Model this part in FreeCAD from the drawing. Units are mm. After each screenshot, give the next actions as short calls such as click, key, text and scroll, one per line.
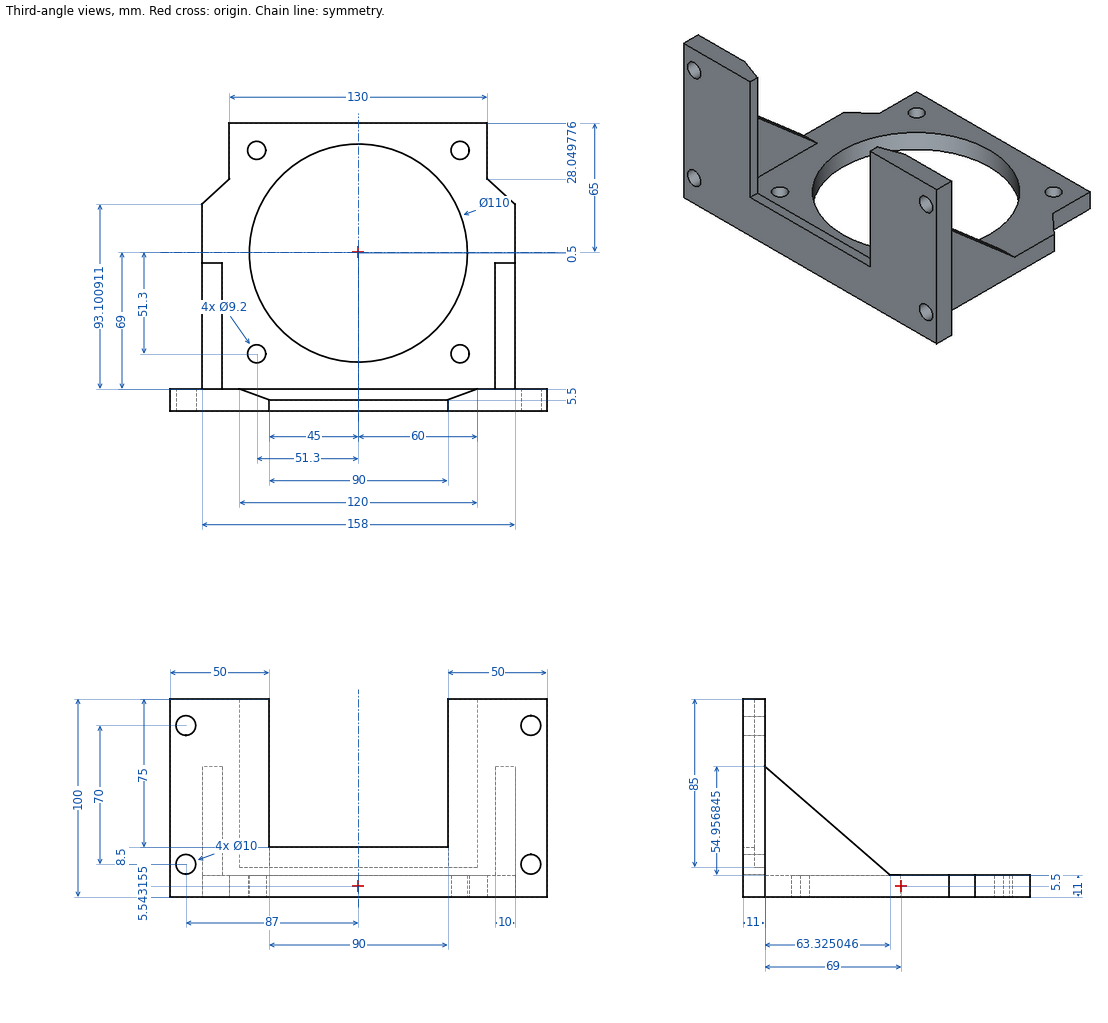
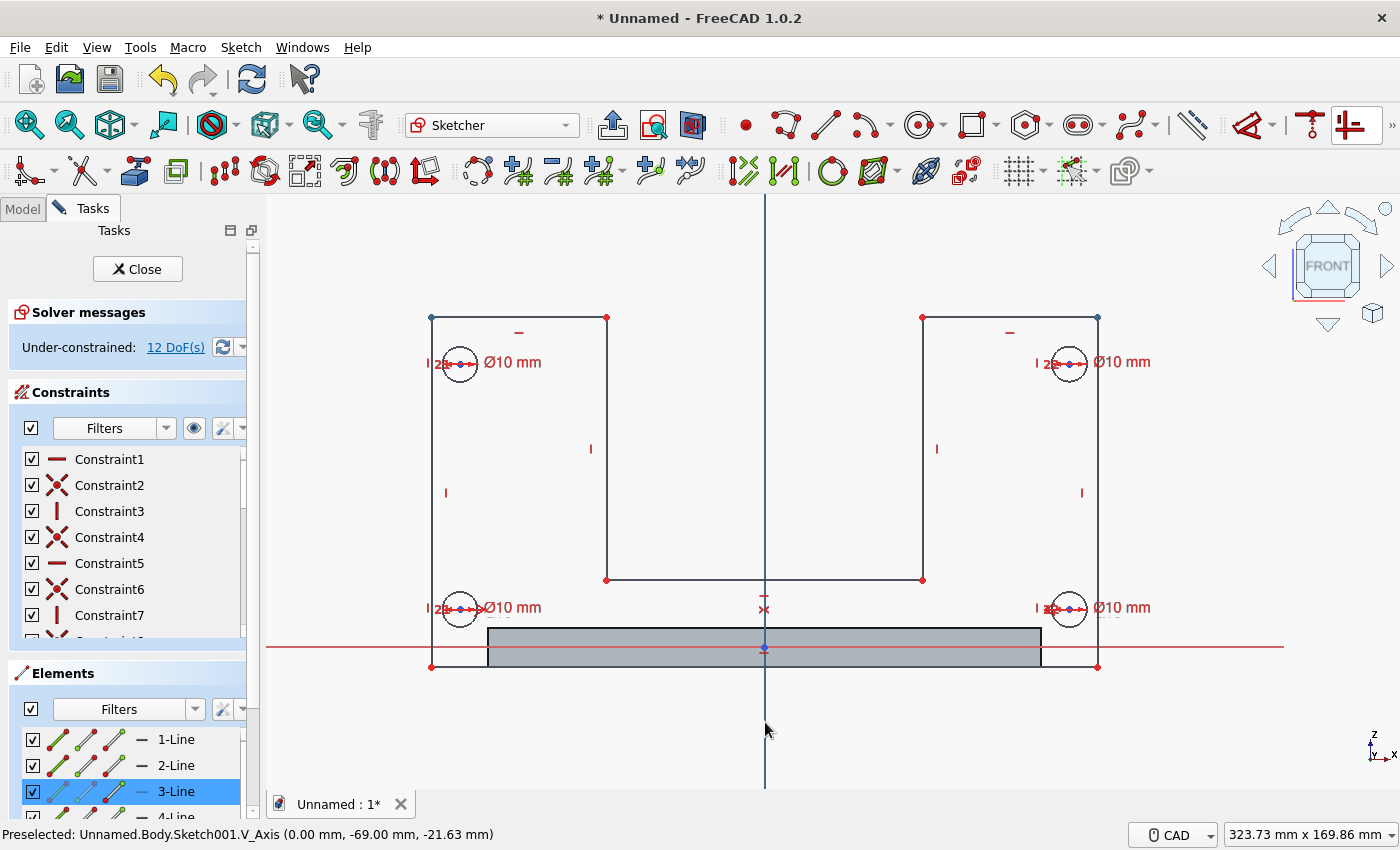
key(s)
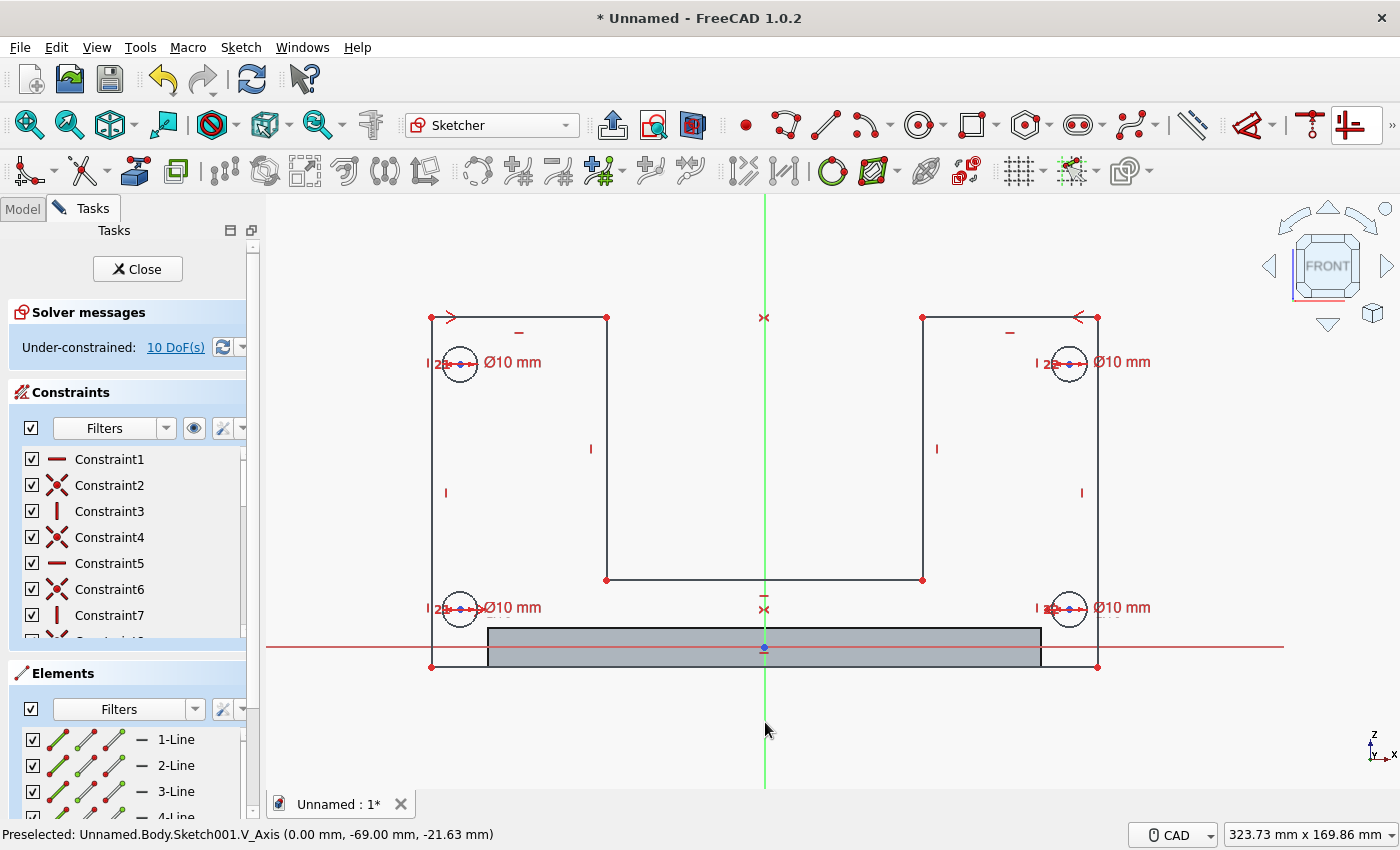
click(1248, 126)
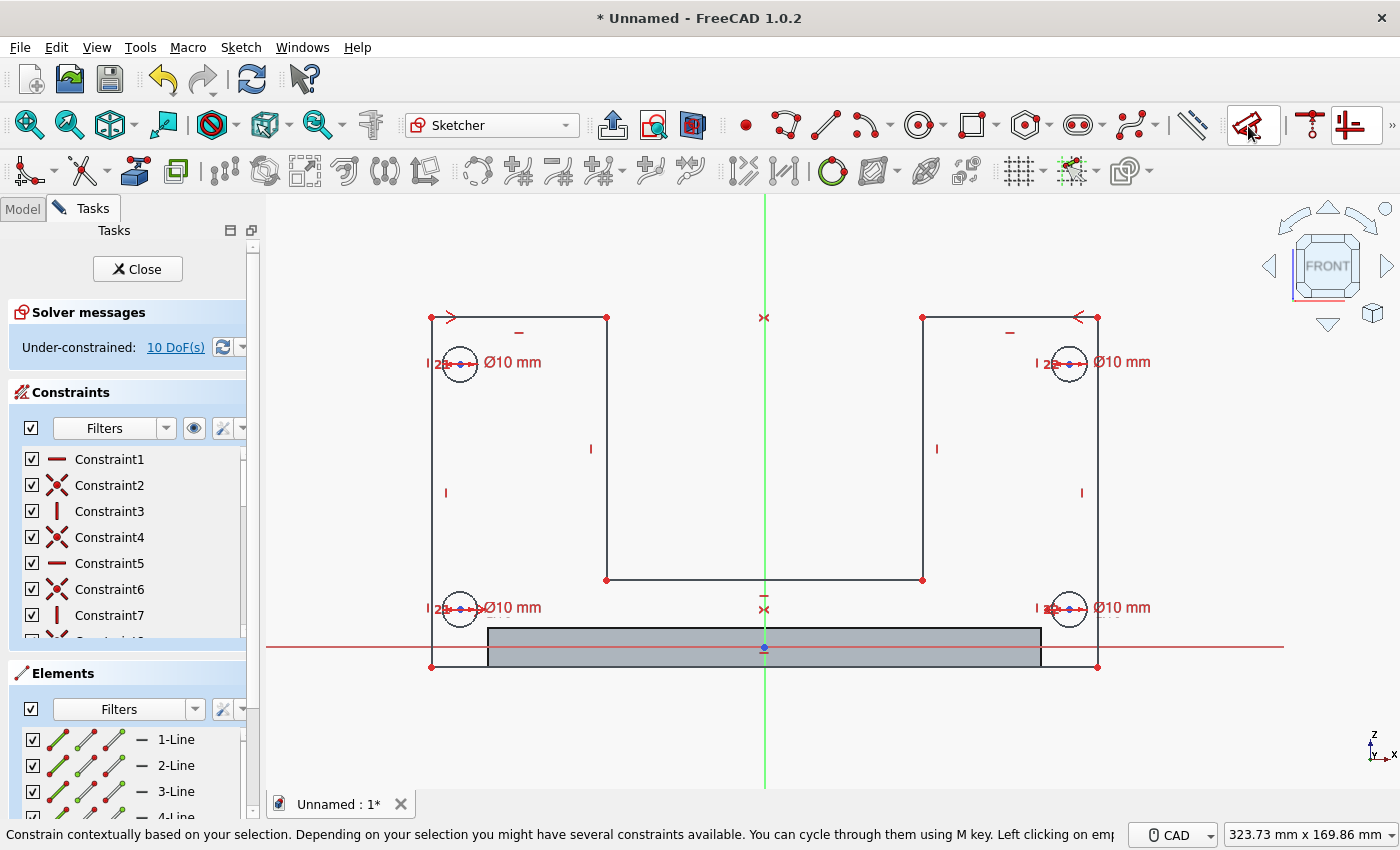
click(828, 580)
click(692, 614)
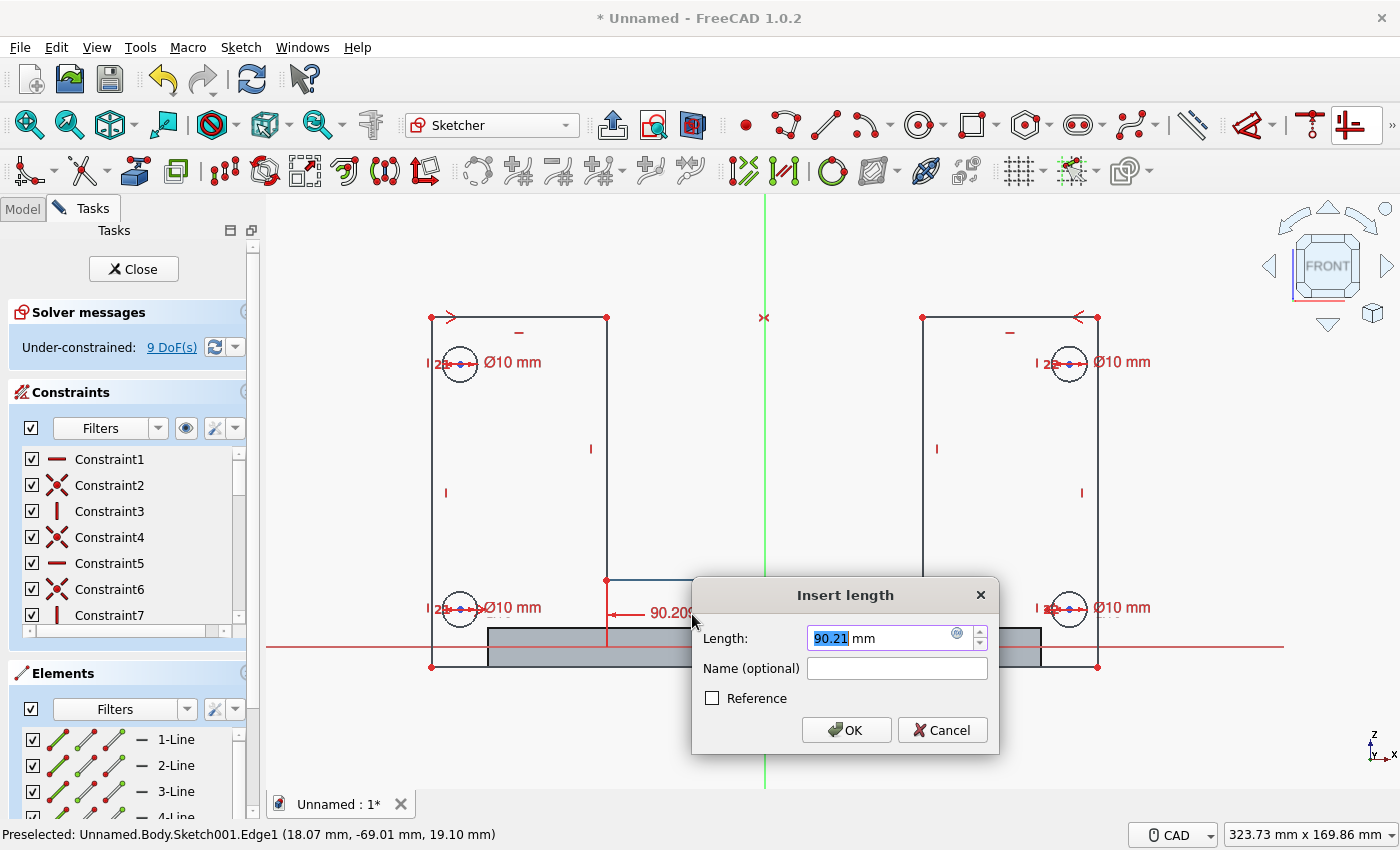
text(90)
key(Return)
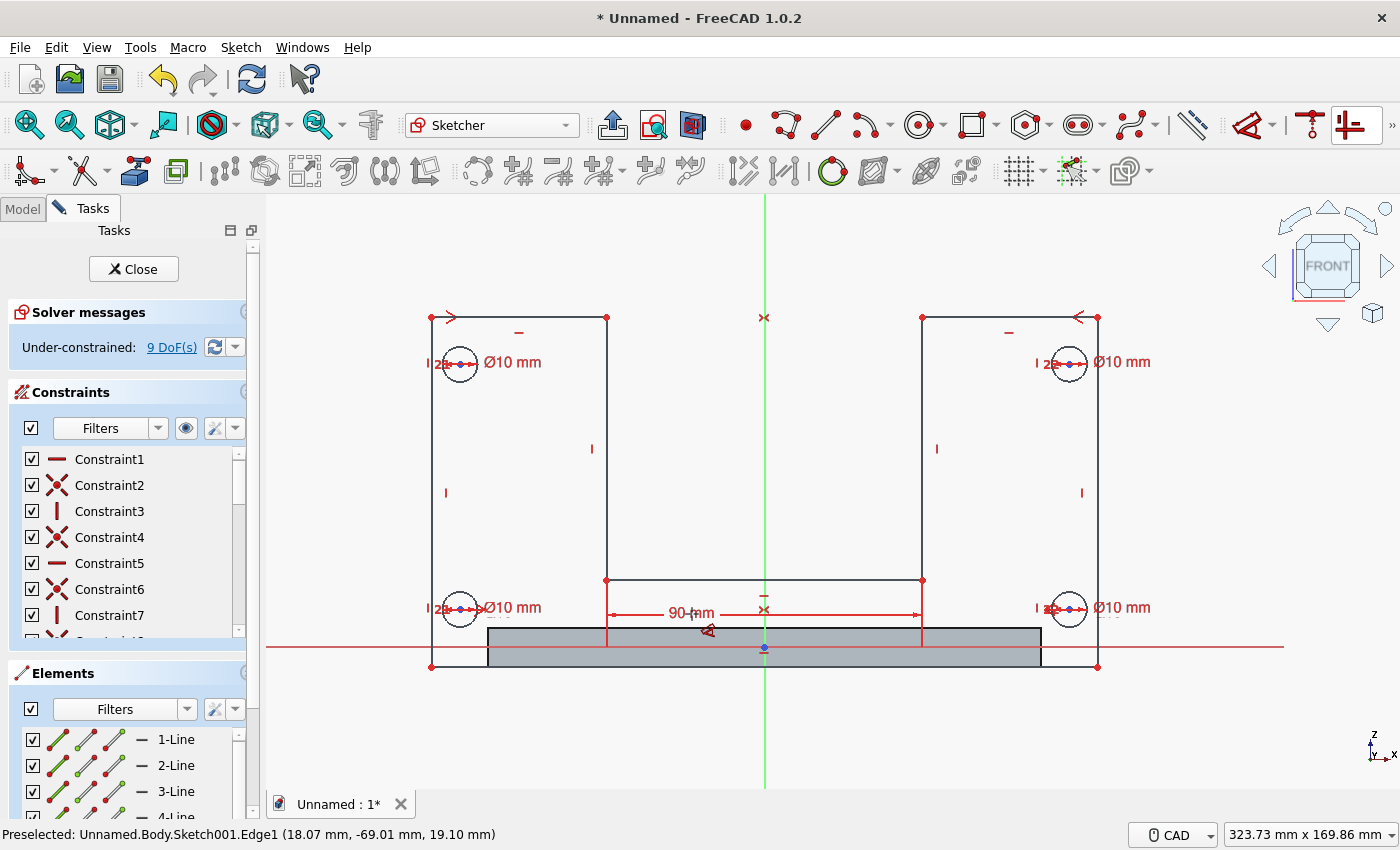
click(607, 501)
click(573, 449)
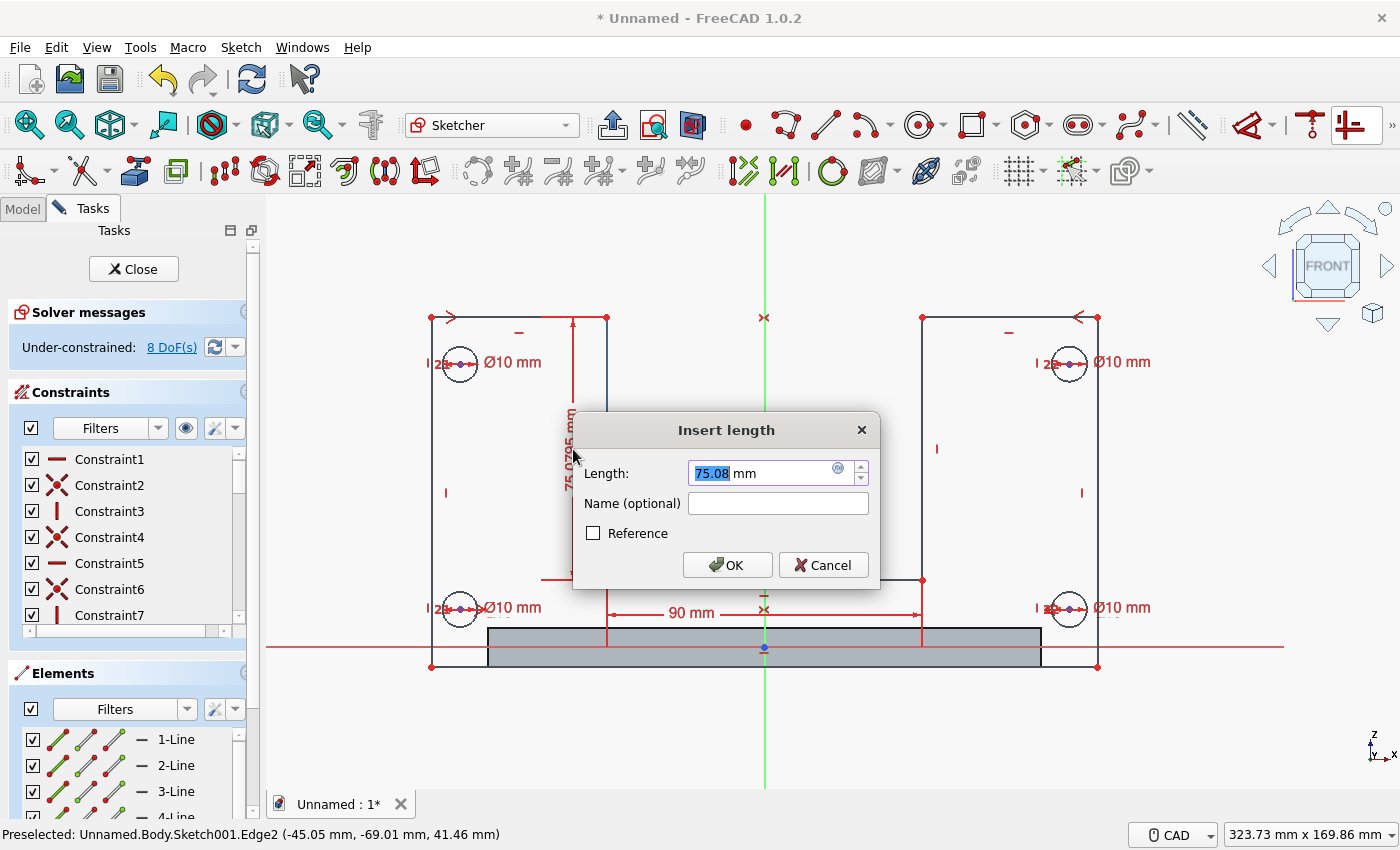
text(75)
key(Return)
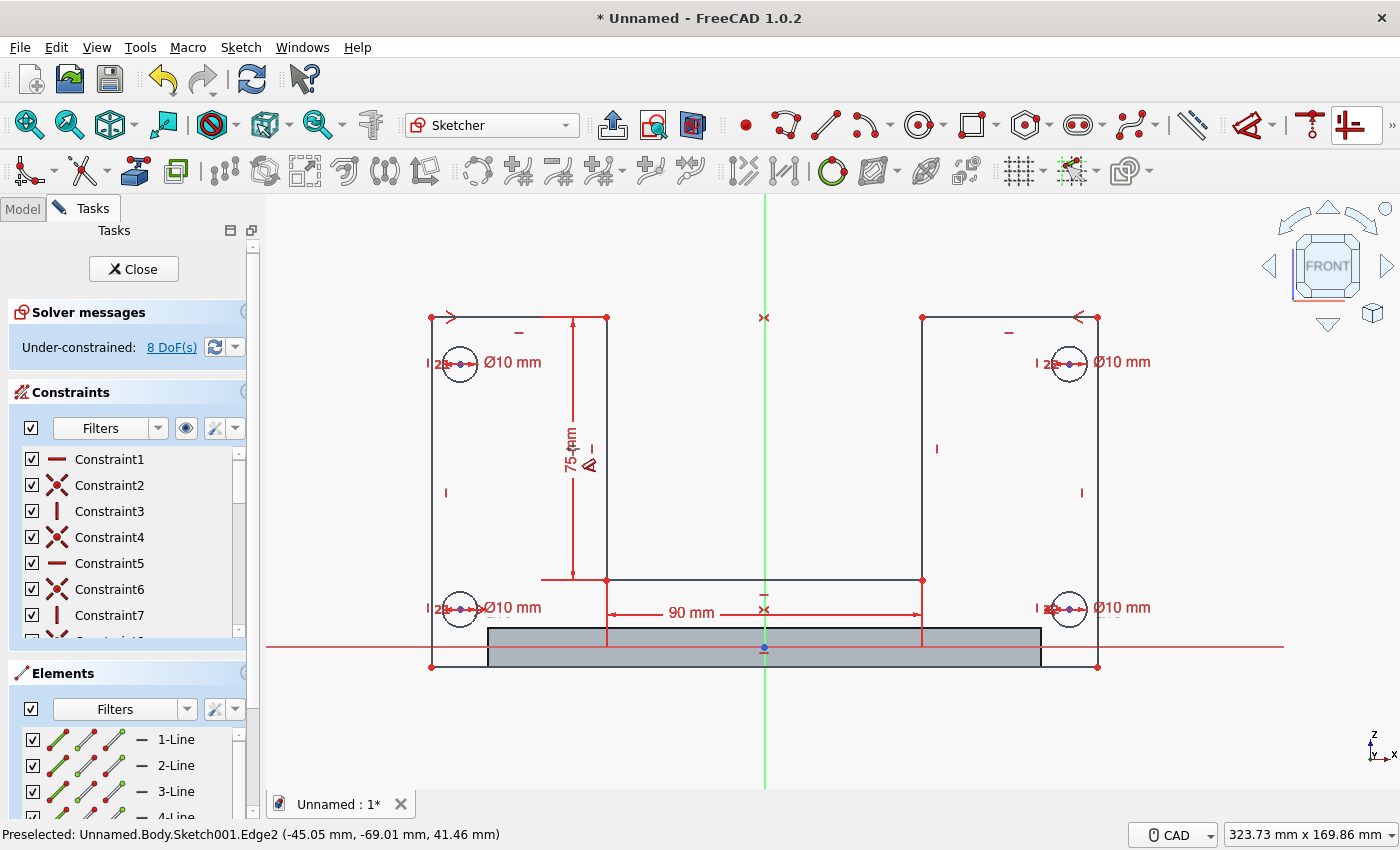
click(554, 317)
click(519, 283)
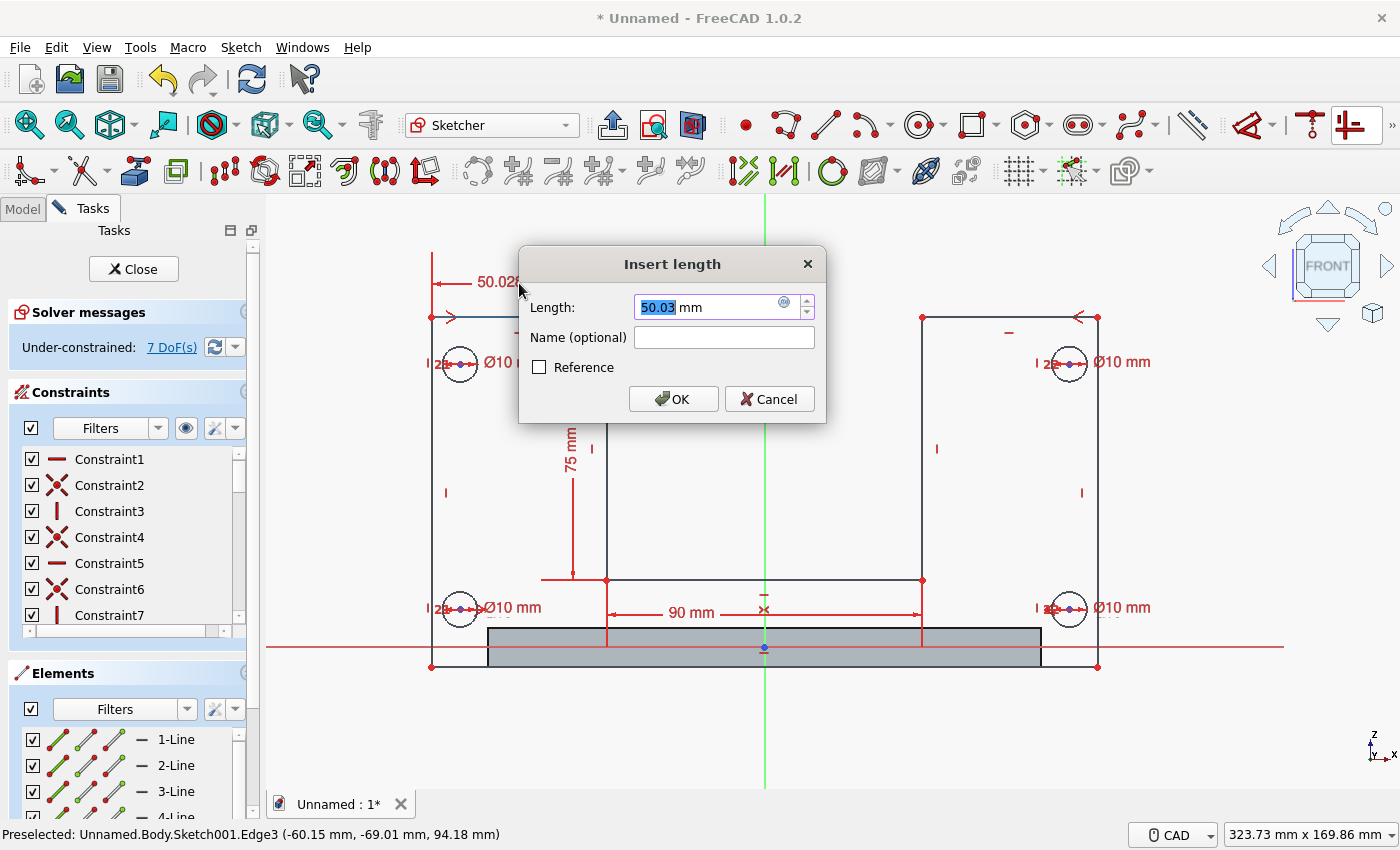
text(50)
key(Return)